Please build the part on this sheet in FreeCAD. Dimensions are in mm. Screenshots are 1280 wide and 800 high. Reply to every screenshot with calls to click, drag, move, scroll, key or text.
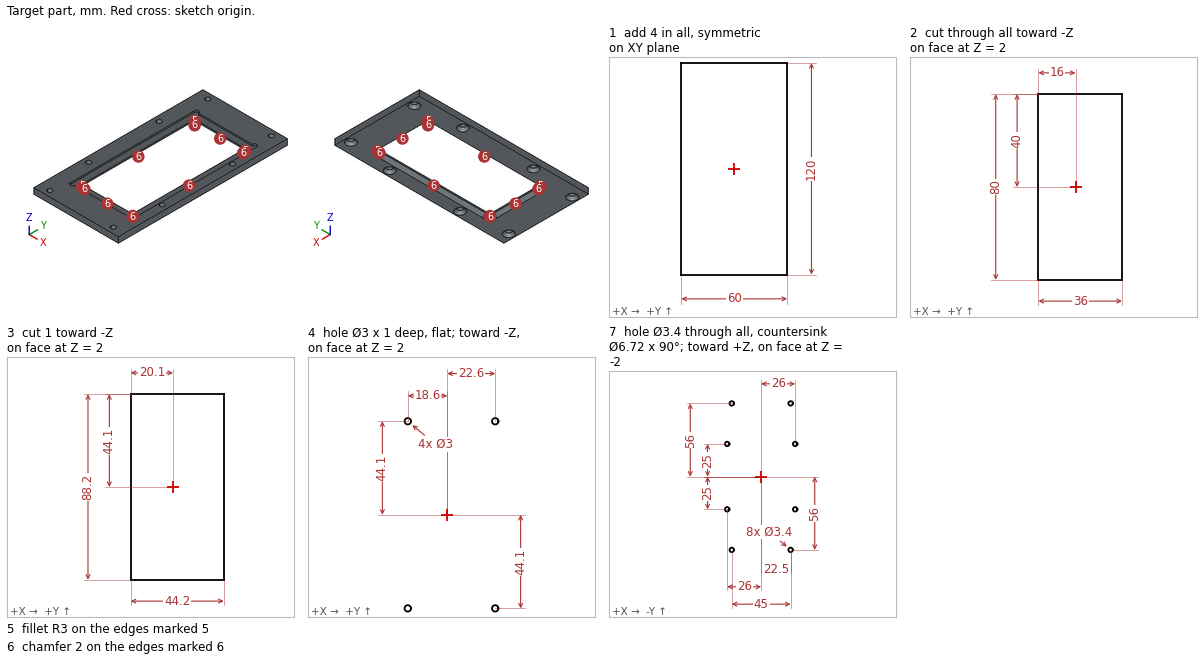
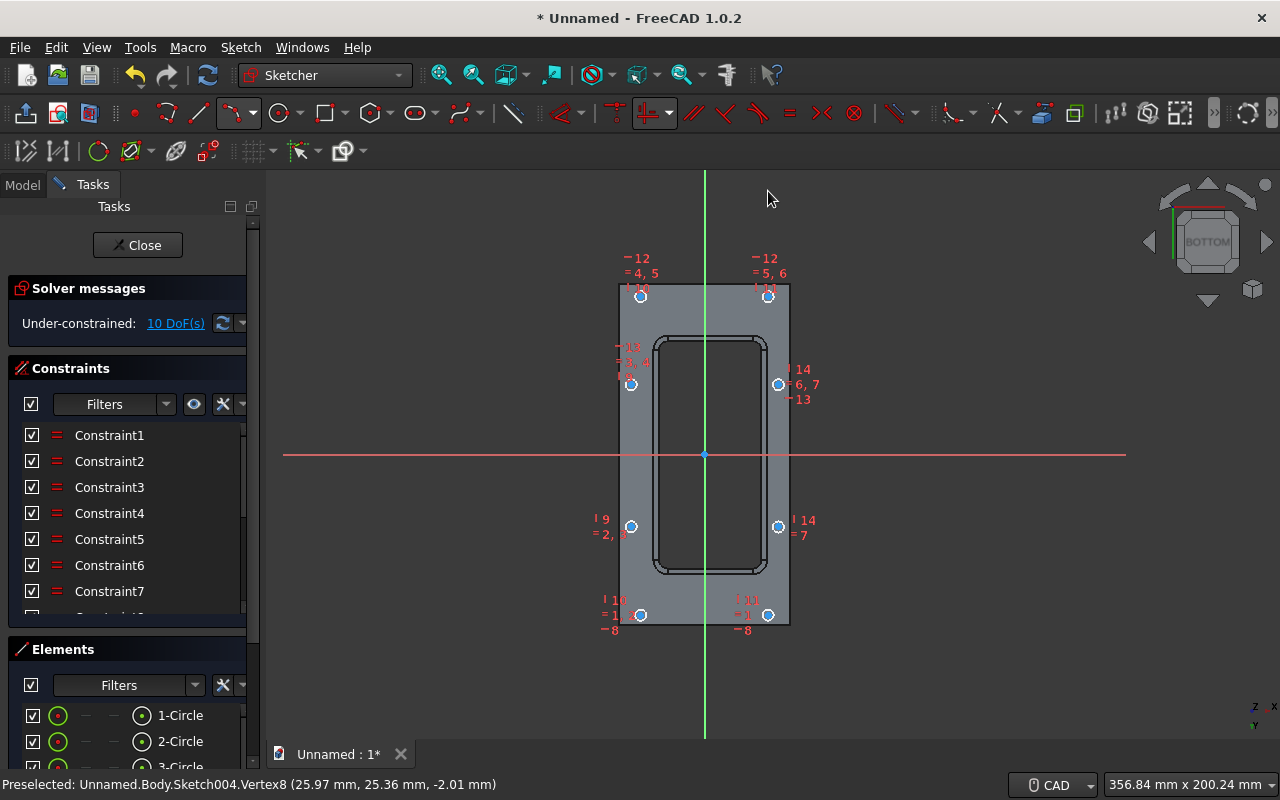
click(631, 527)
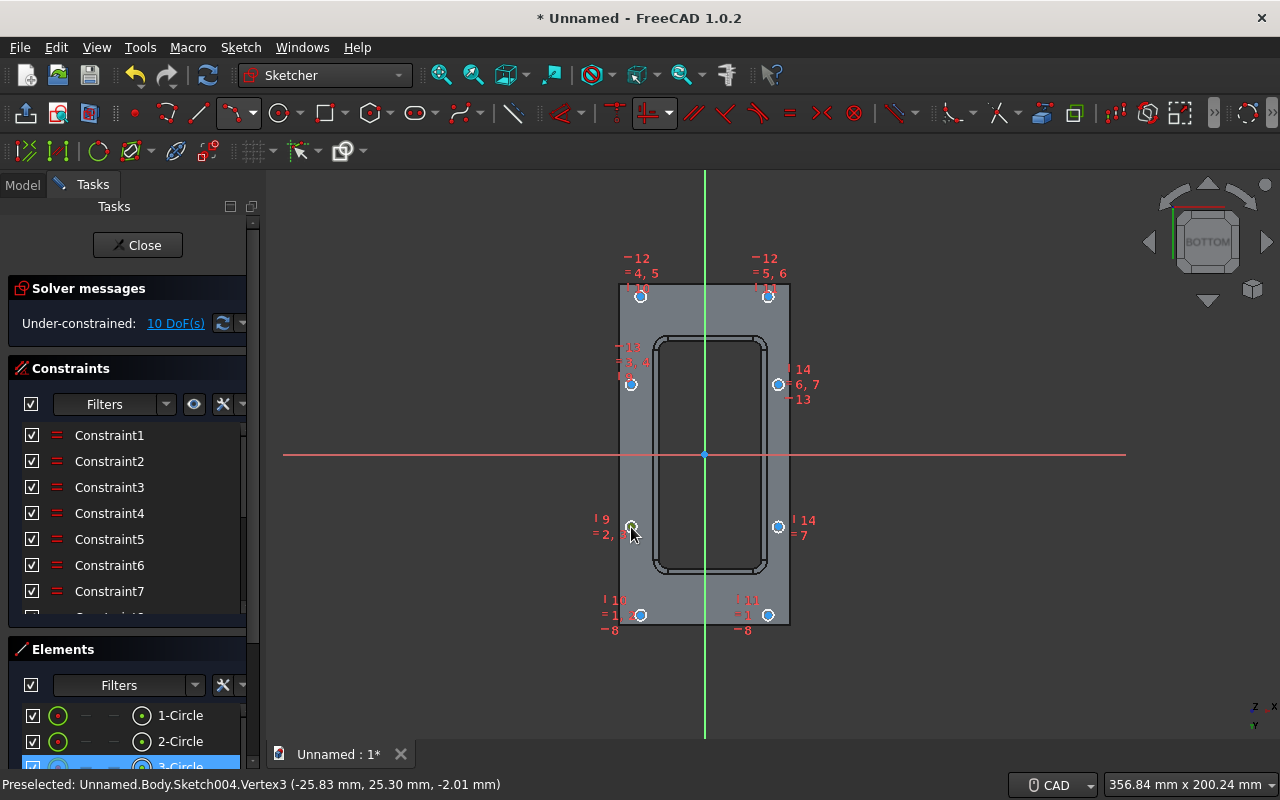
click(778, 527)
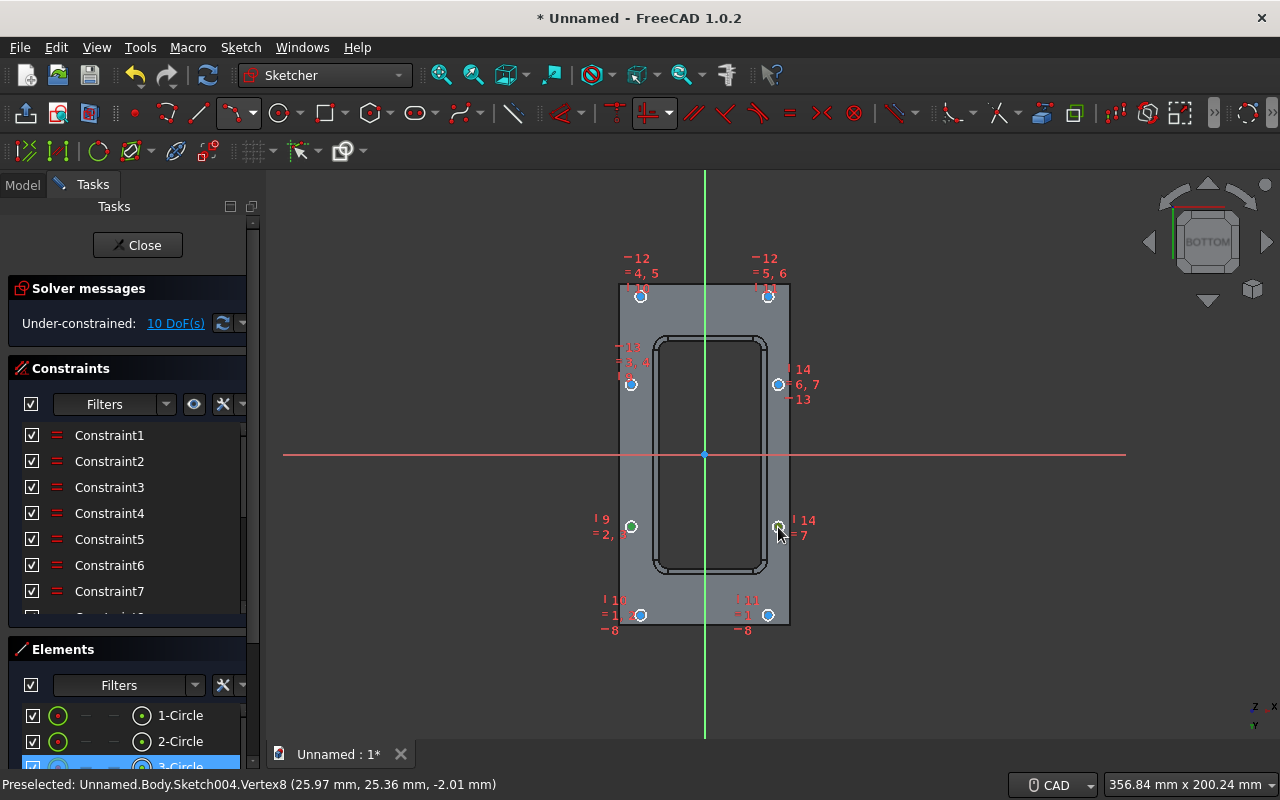
key(h)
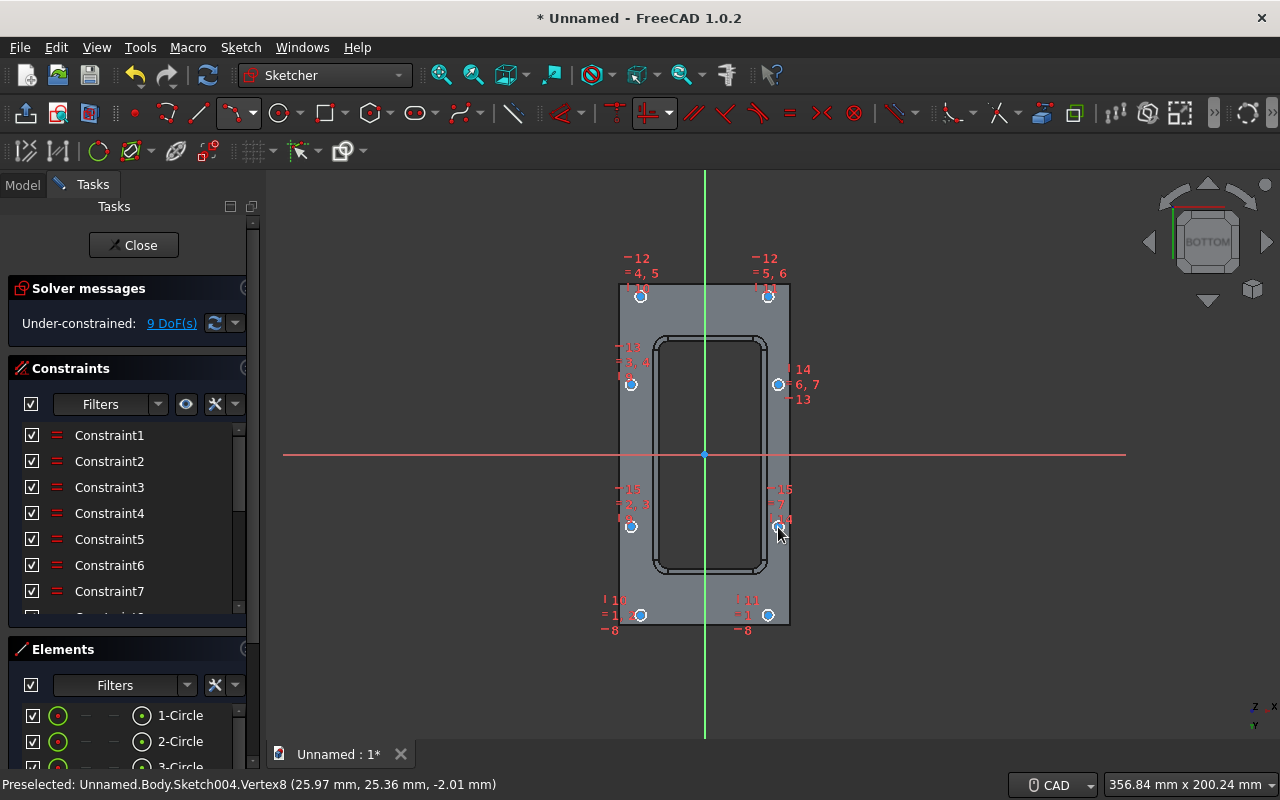
click(560, 114)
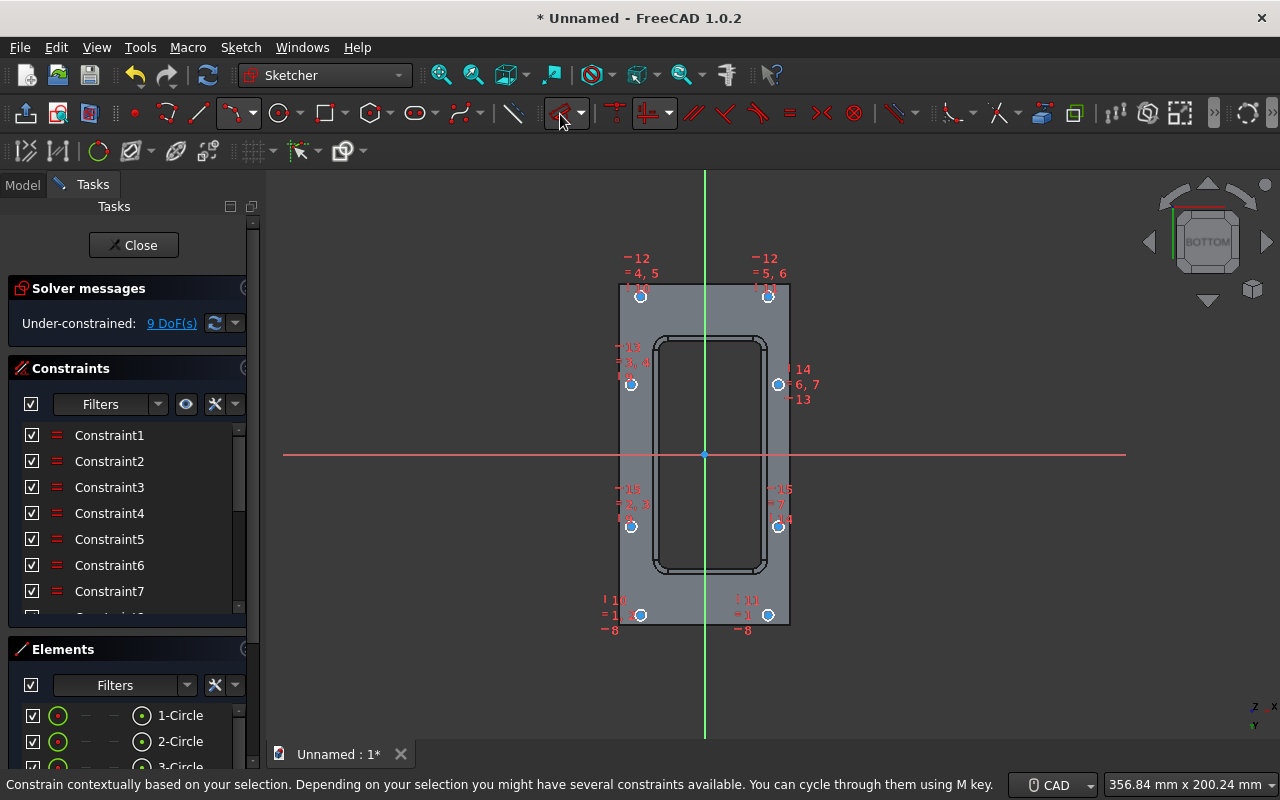
scroll(774, 615, up, 8)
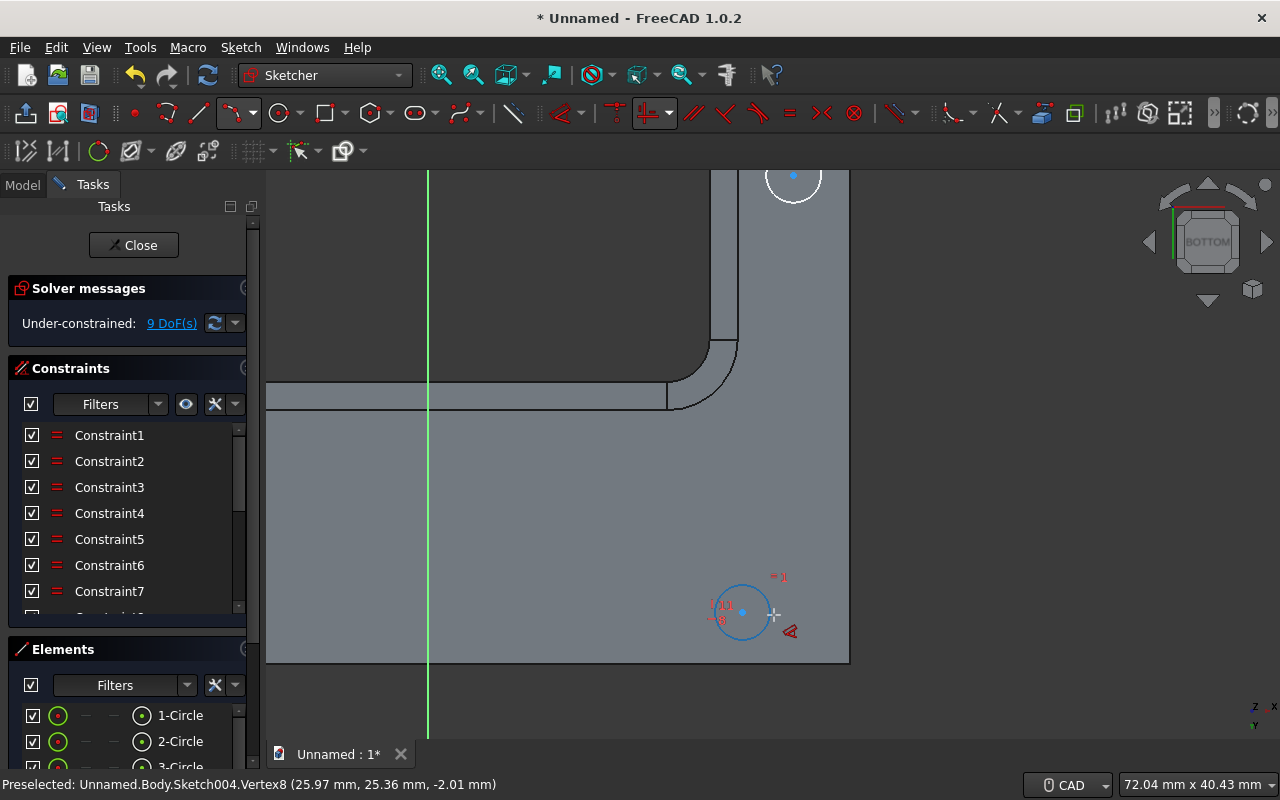
click(770, 613)
click(802, 614)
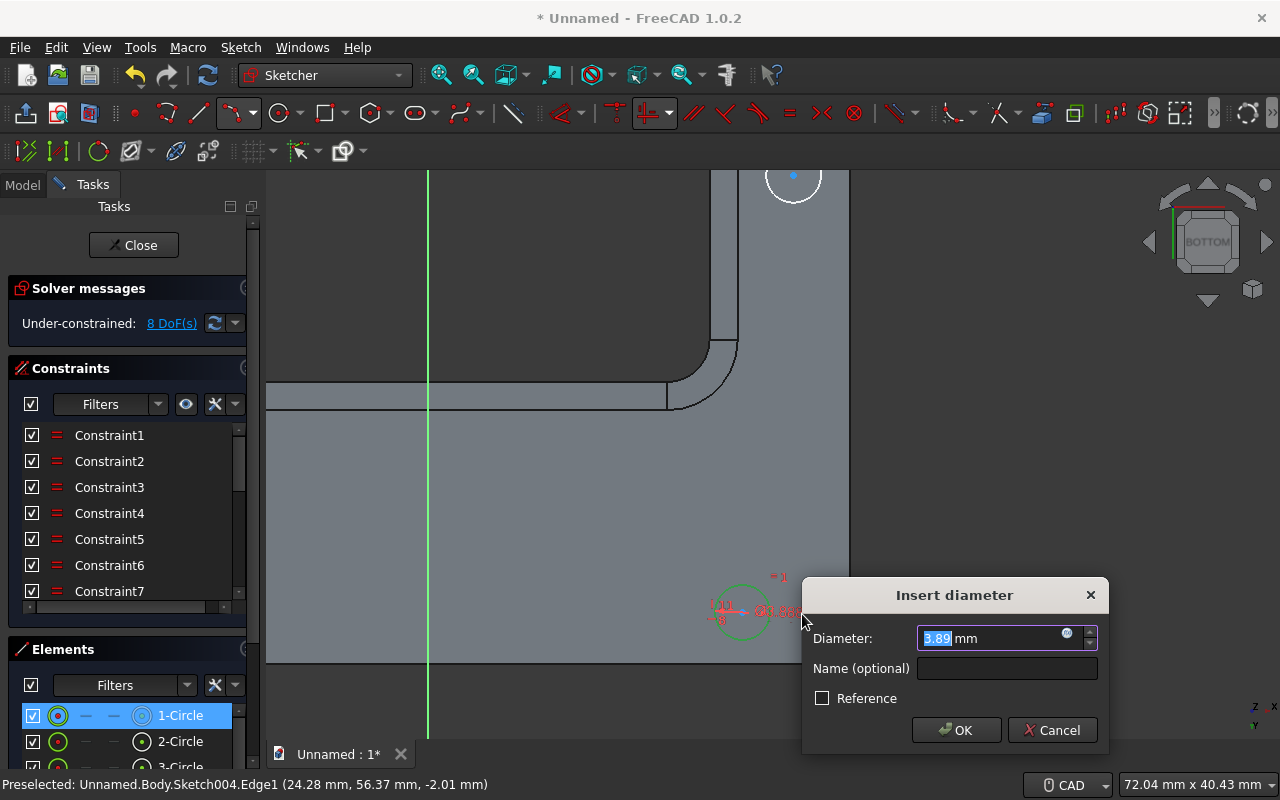
text(3.4)
key(Return)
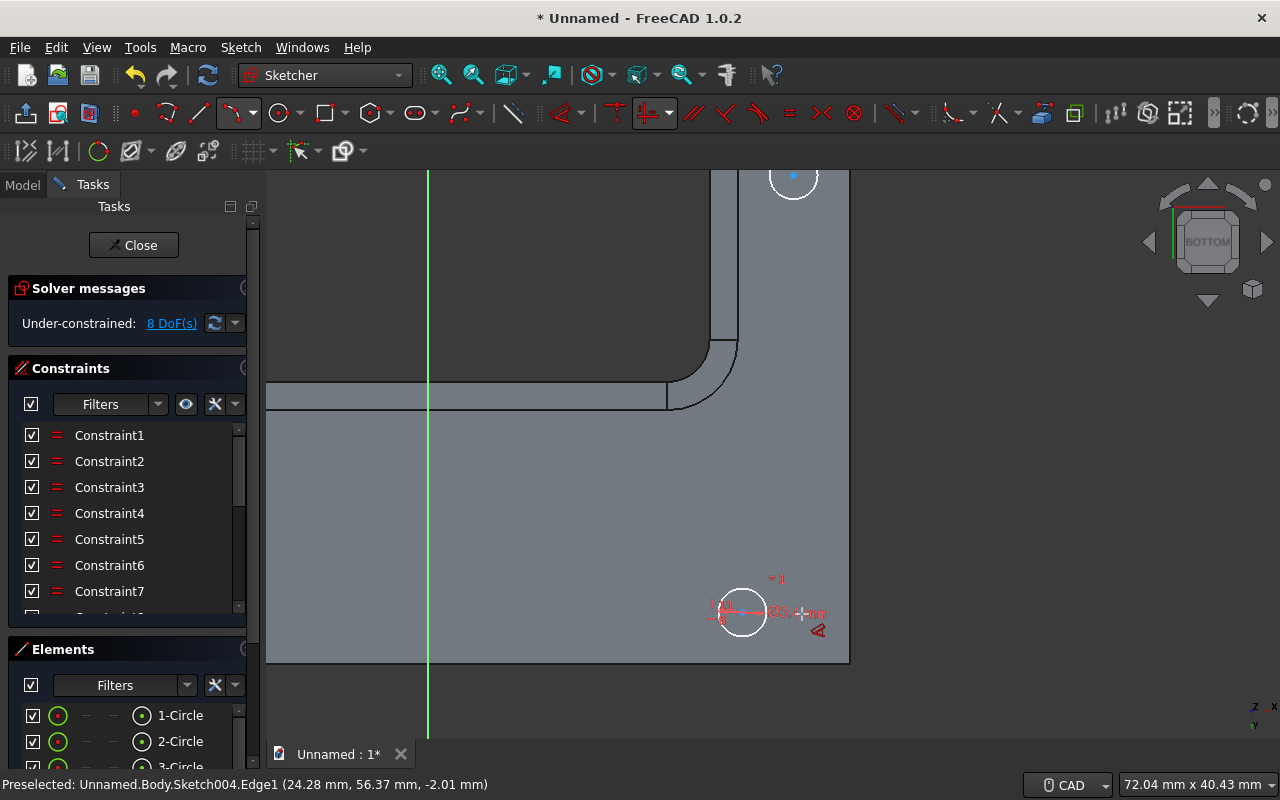
scroll(774, 615, down, 8)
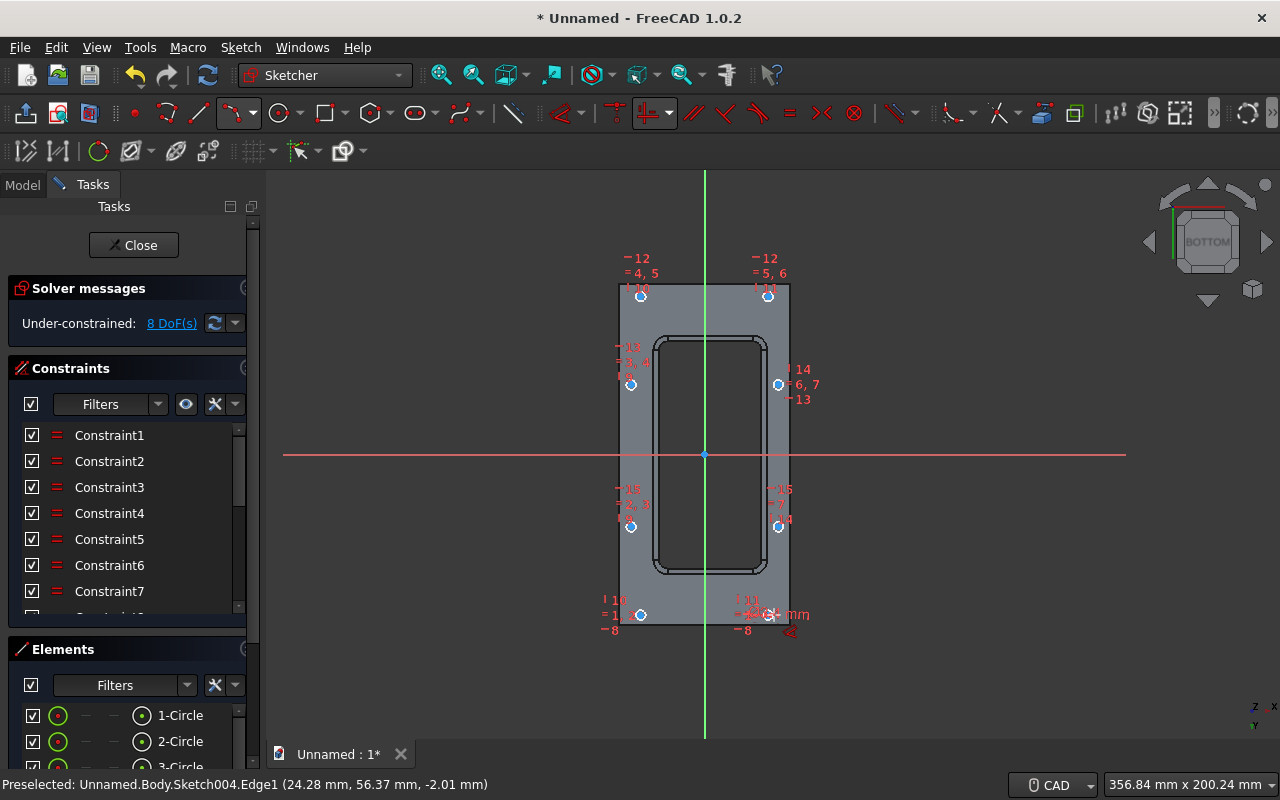
click(768, 615)
click(802, 535)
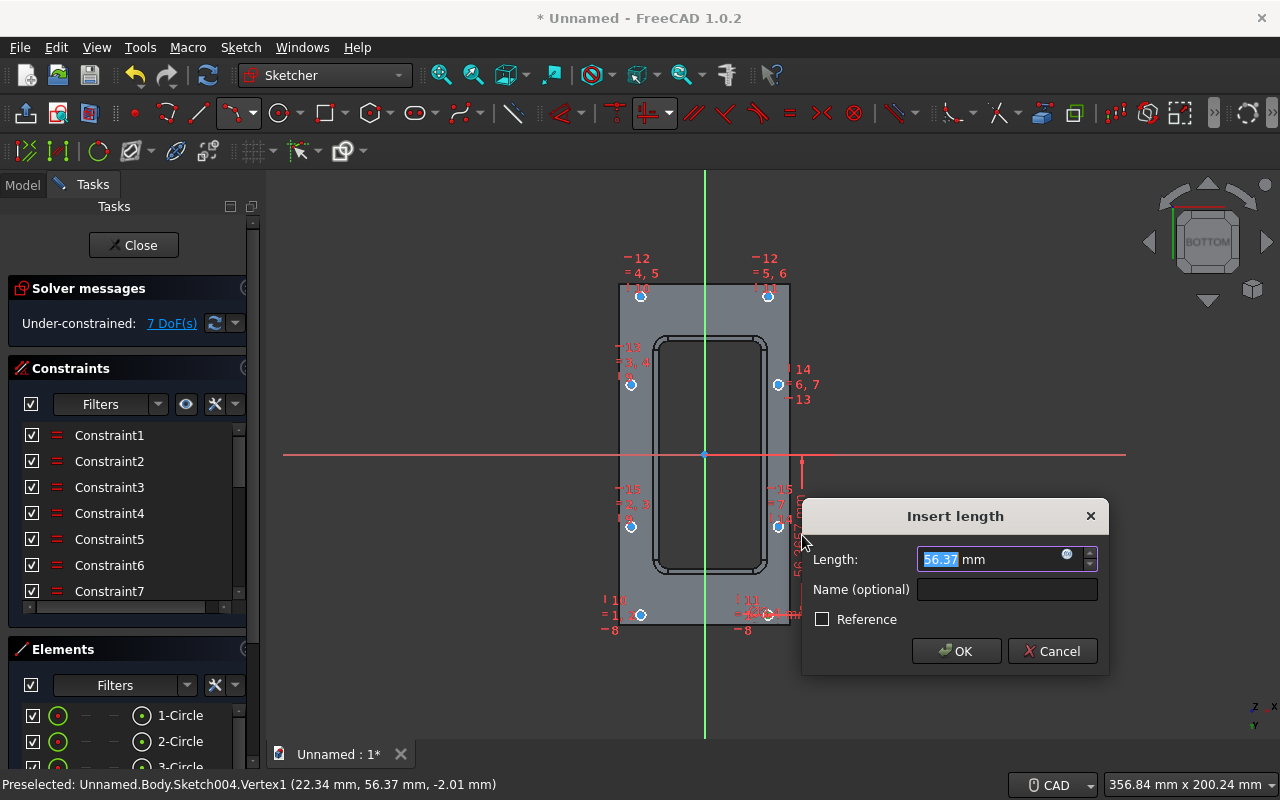
text(56)
key(Return)